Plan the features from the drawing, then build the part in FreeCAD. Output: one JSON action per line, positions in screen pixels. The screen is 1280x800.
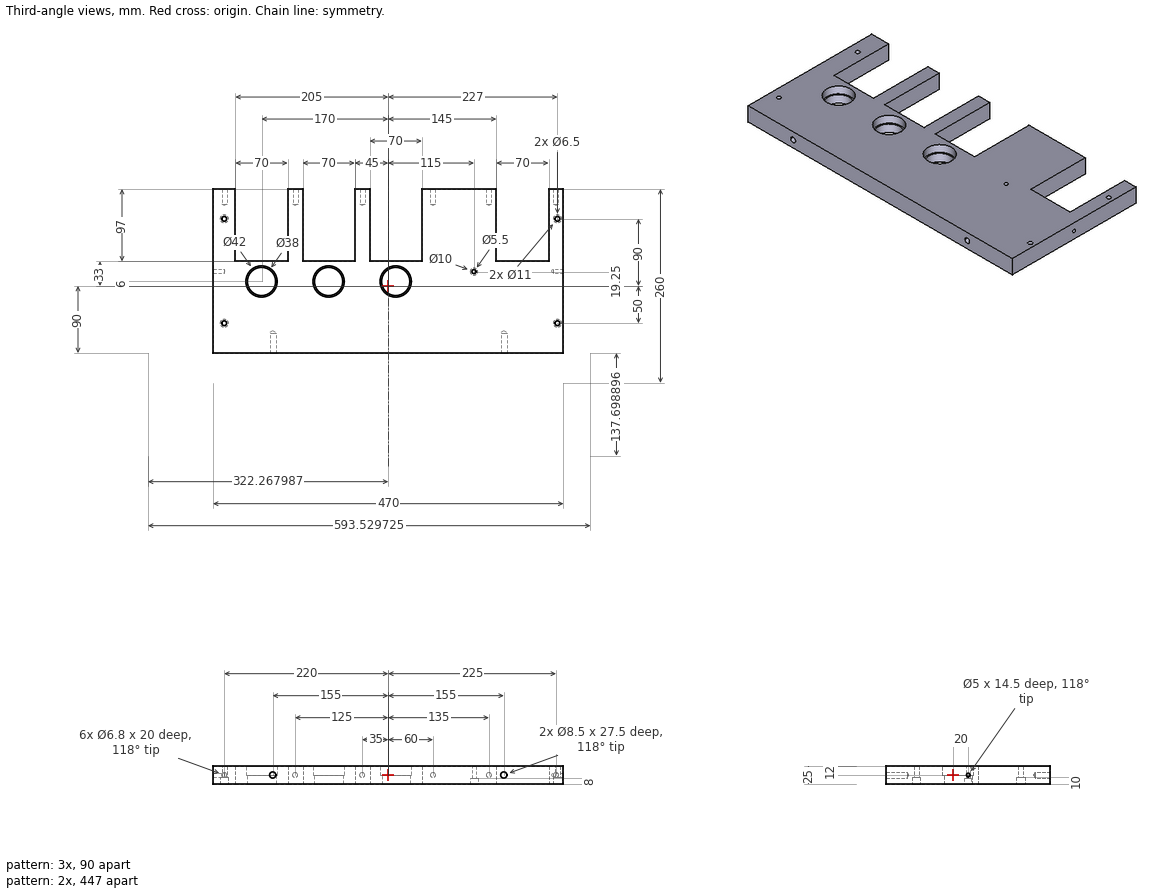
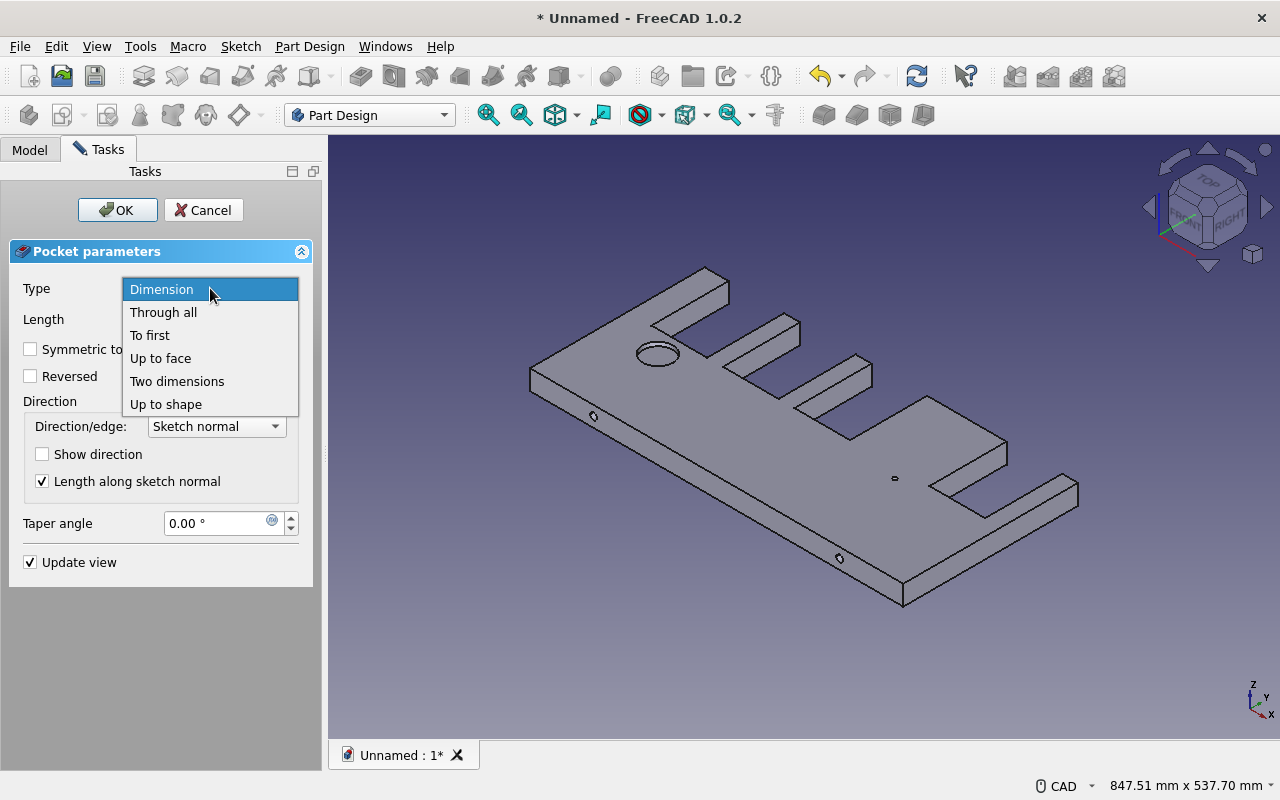
{"action": "left_click", "coordinate": [208, 312]}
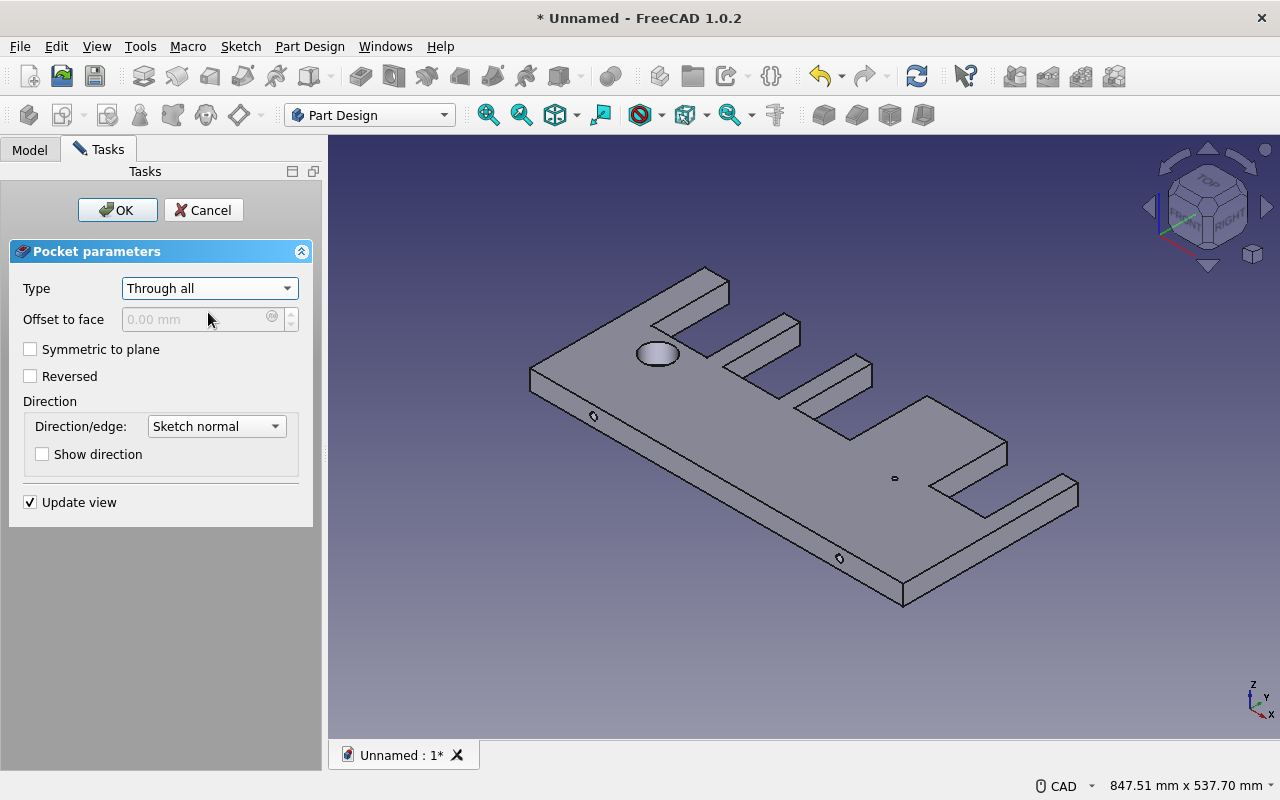
{"action": "left_click", "coordinate": [118, 210]}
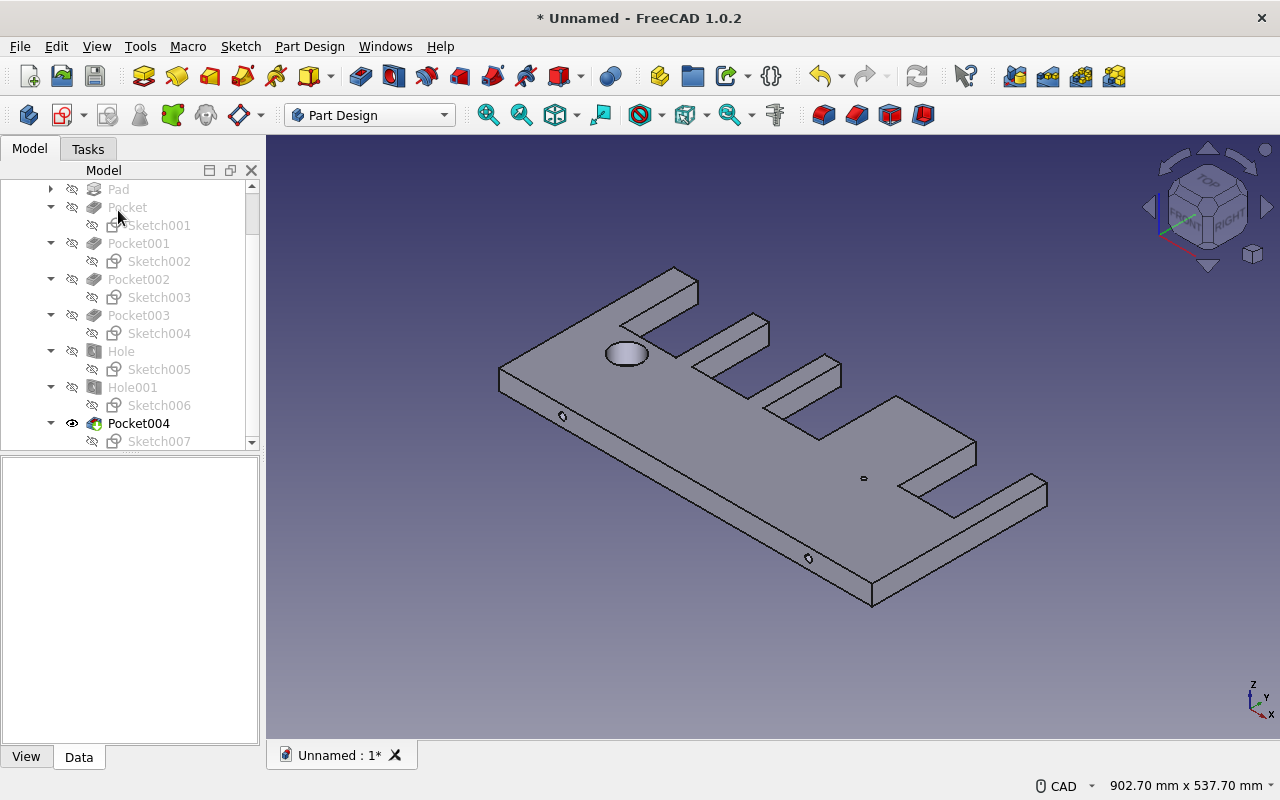
{"action": "left_click", "coordinate": [801, 470]}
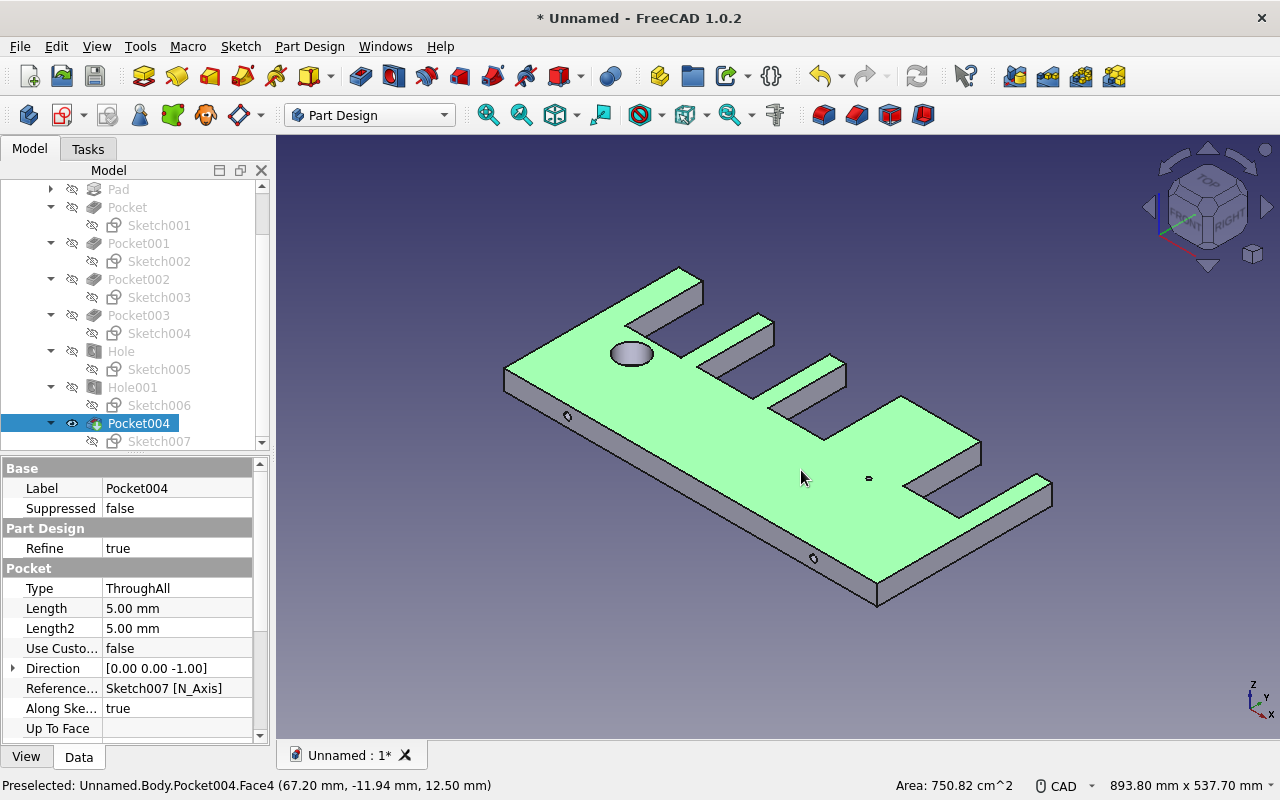
{"action": "left_click", "coordinate": [62, 116]}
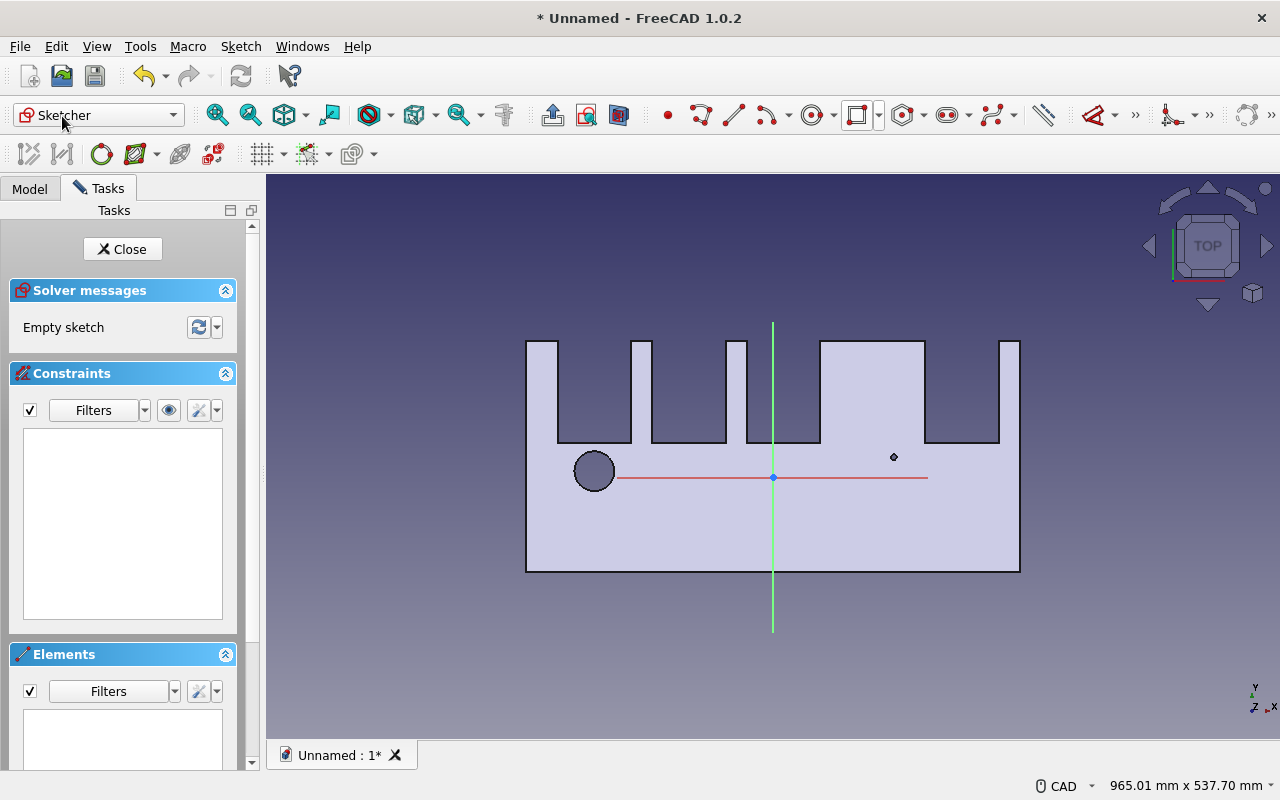
{"action": "scroll", "coordinate": [577, 474], "scroll_direction": "up", "scroll_amount": 10}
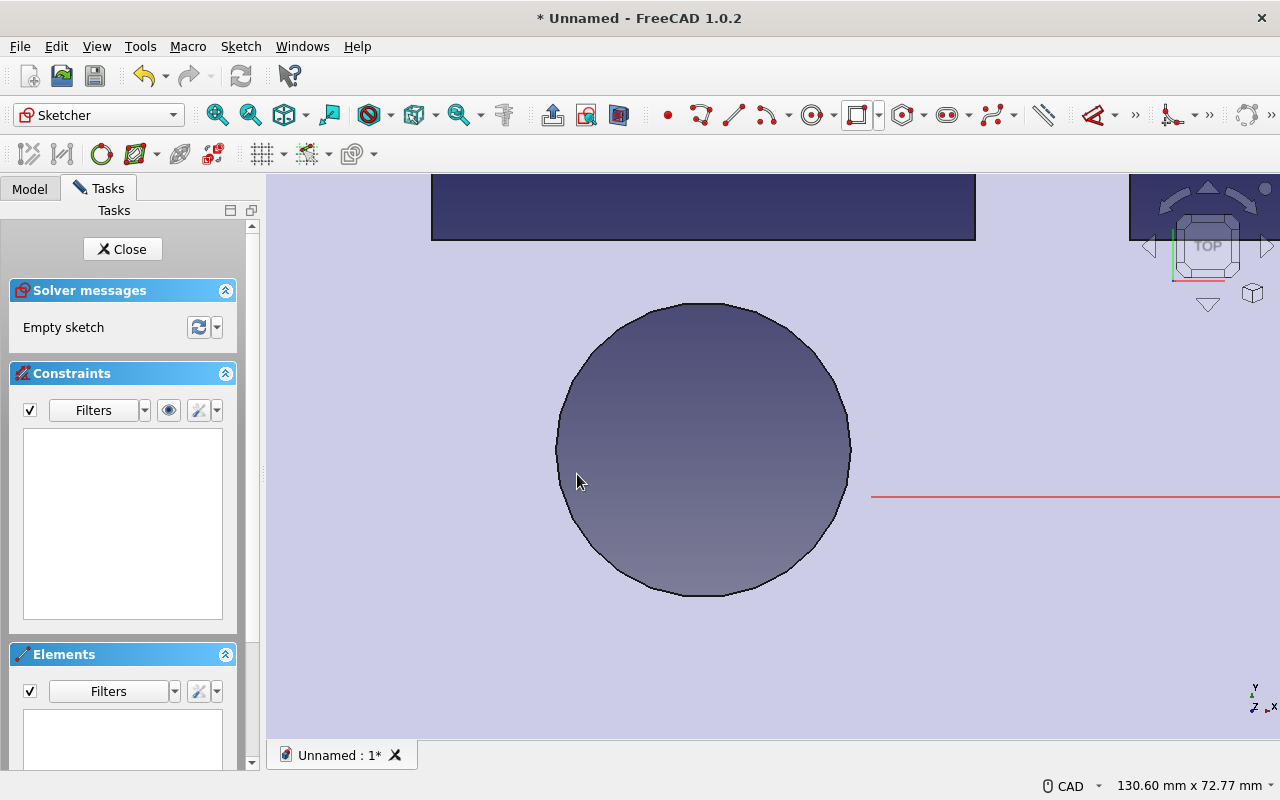
{"action": "left_click", "coordinate": [812, 116]}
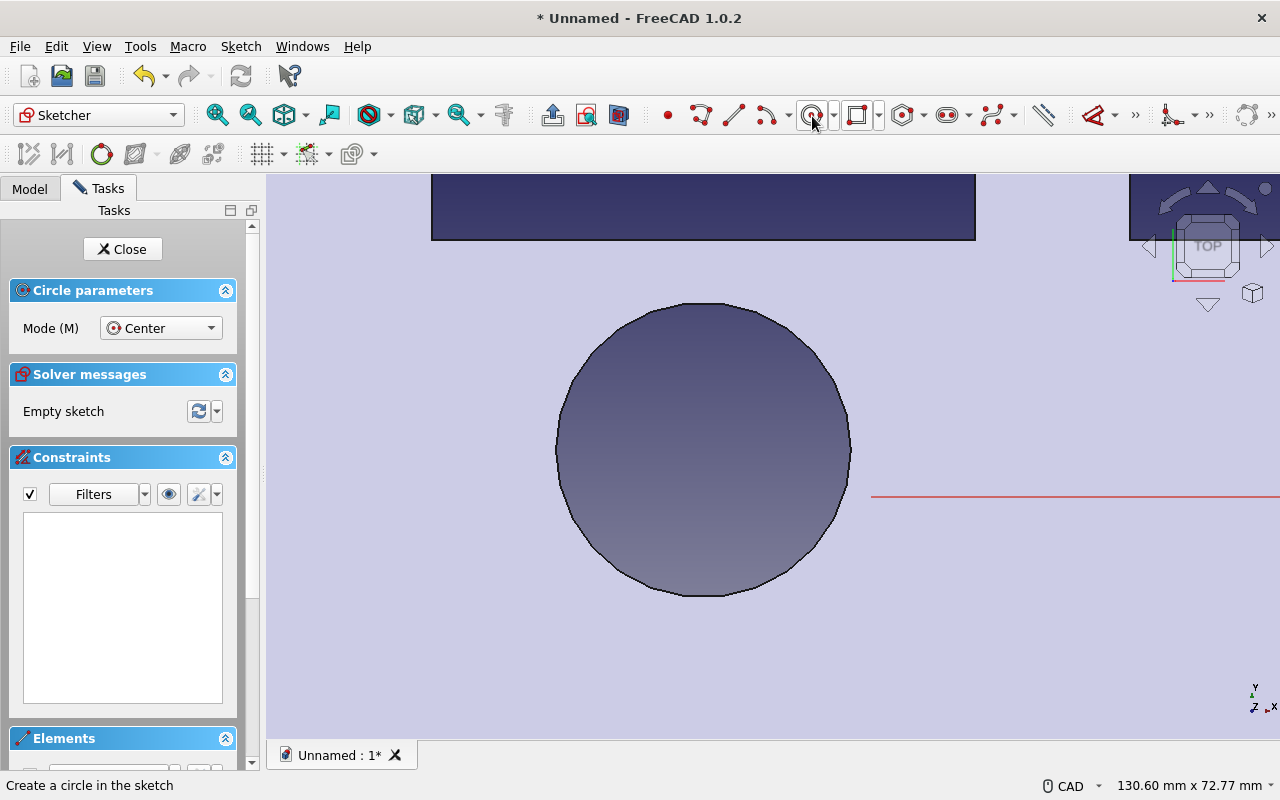
{"action": "left_click", "coordinate": [703, 450]}
{"action": "mouse_move", "coordinate": [819, 335]}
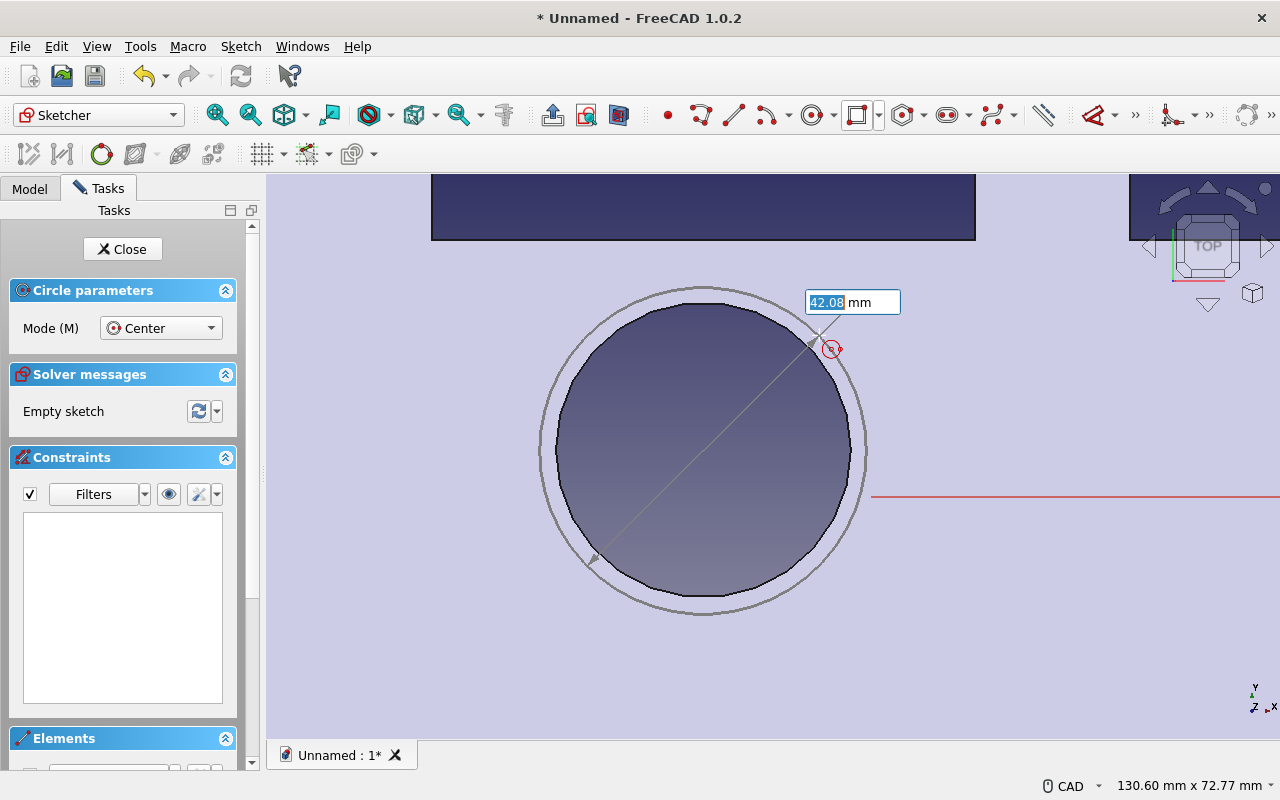
{"action": "type", "text": "42"}
{"action": "key", "text": "Return"}
{"action": "key", "text": "Escape"}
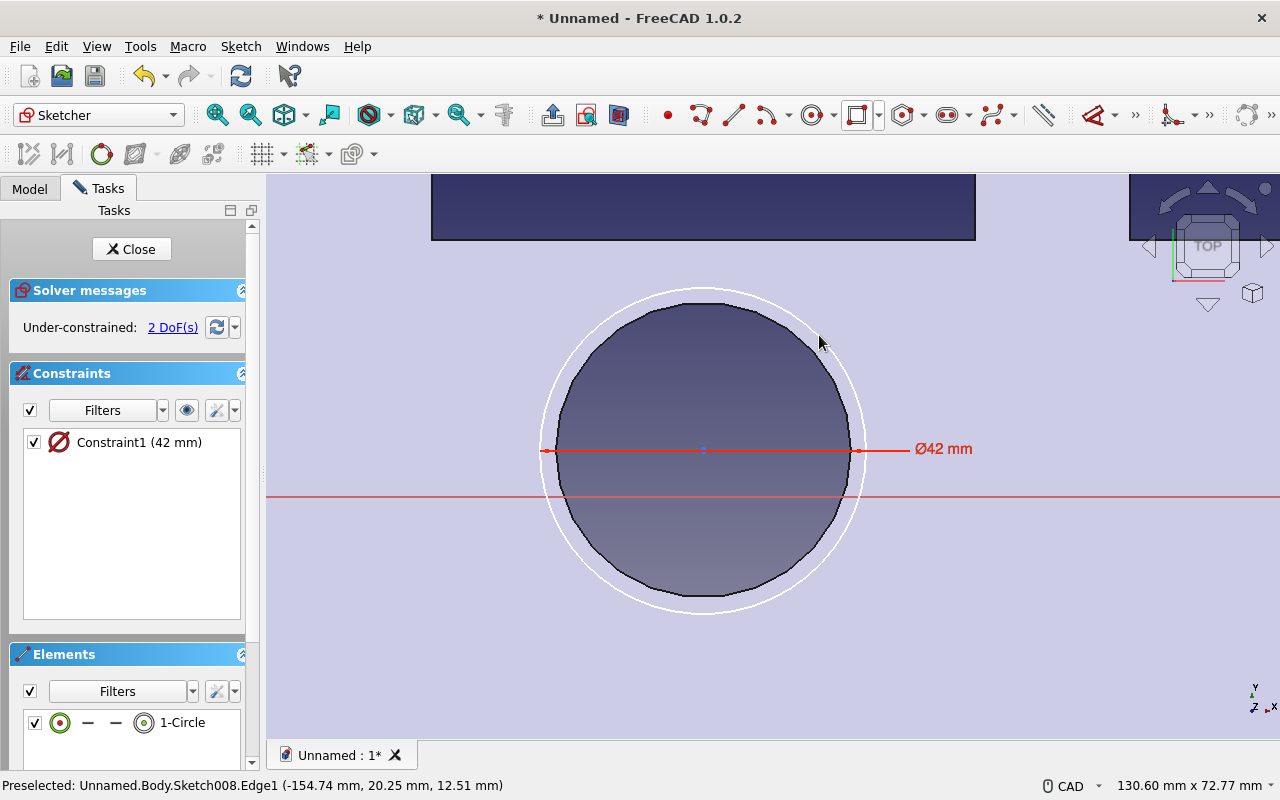
{"action": "left_click", "coordinate": [1092, 116]}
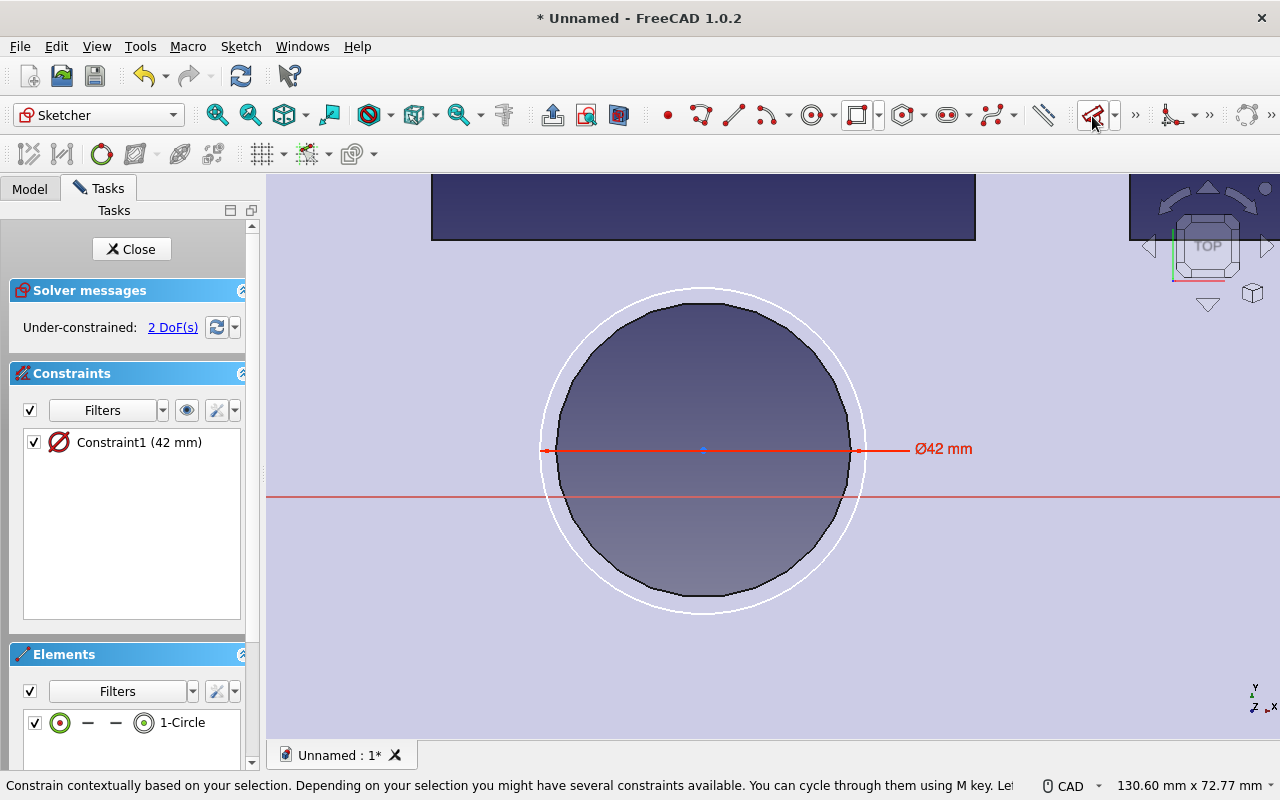
{"action": "left_click", "coordinate": [703, 451]}
{"action": "left_click", "coordinate": [669, 474]}